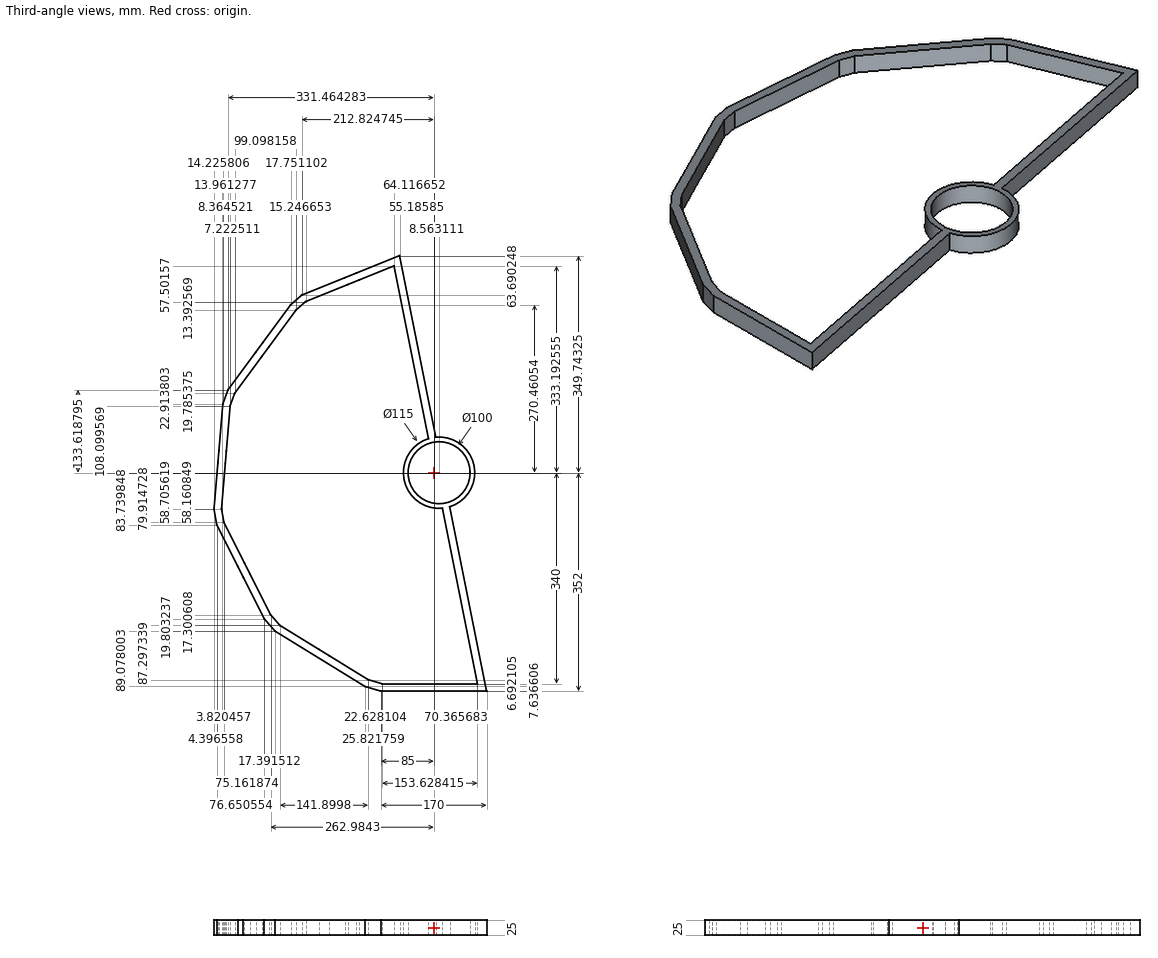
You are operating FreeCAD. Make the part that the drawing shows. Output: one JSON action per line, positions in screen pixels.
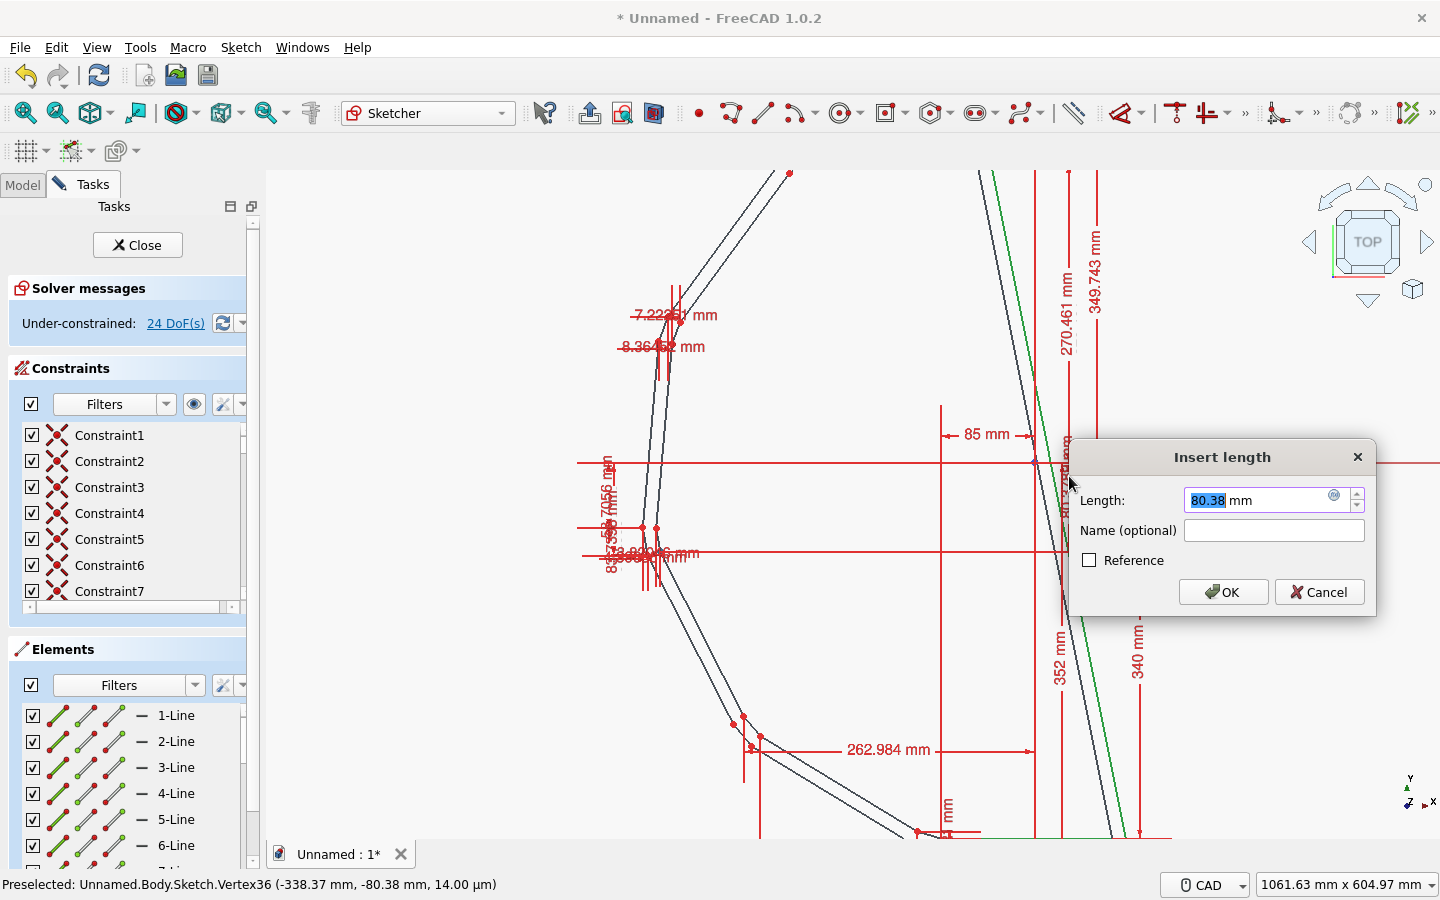
{"action": "type", "text": "79.914728"}
{"action": "key", "text": "Return"}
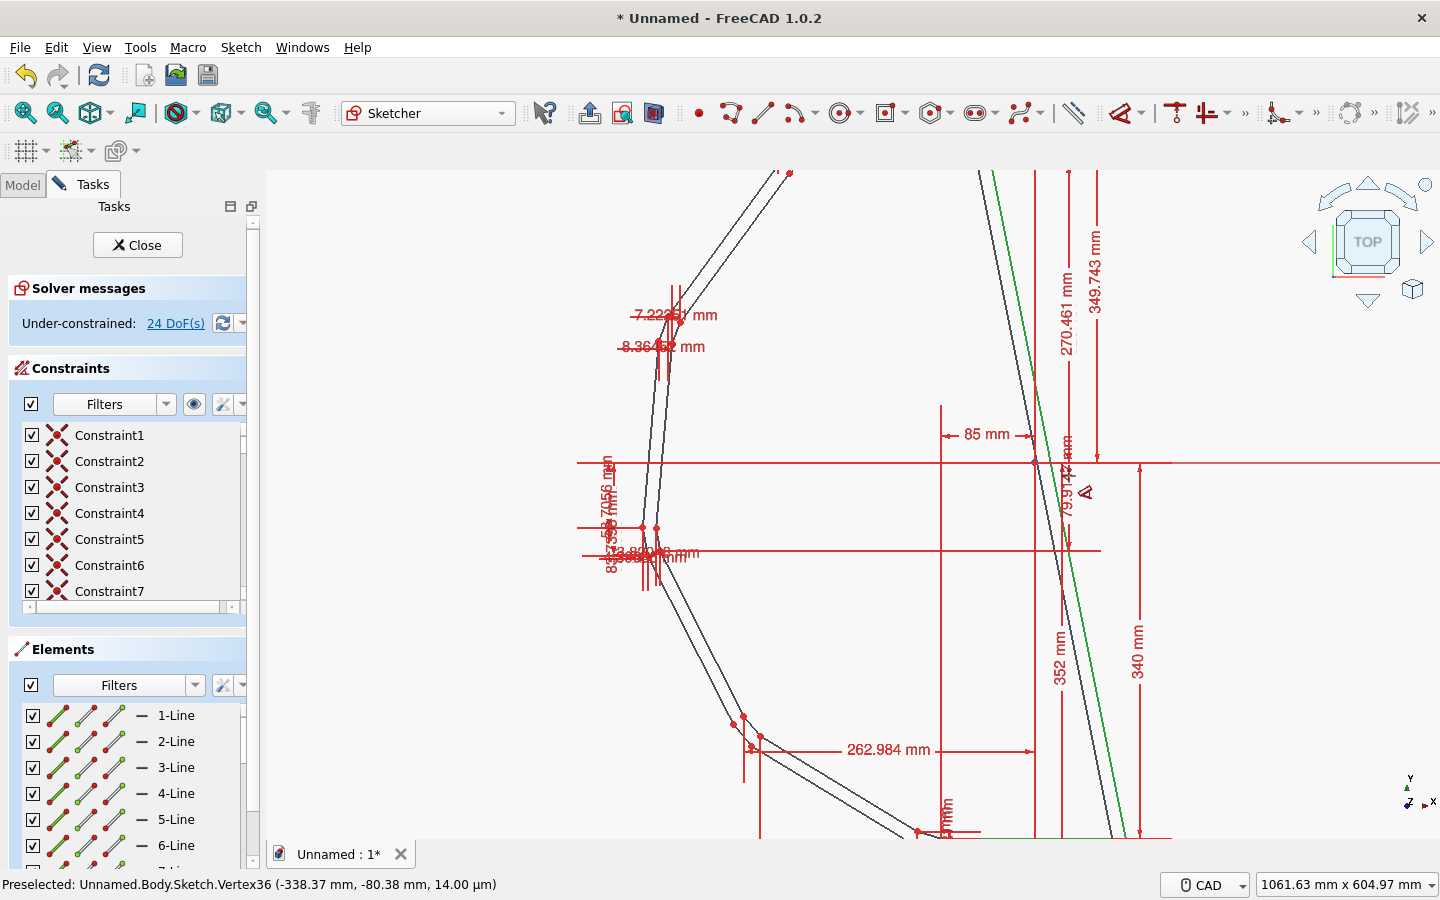
{"action": "left_click", "coordinate": [656, 528]}
{"action": "left_click", "coordinate": [1093, 511]}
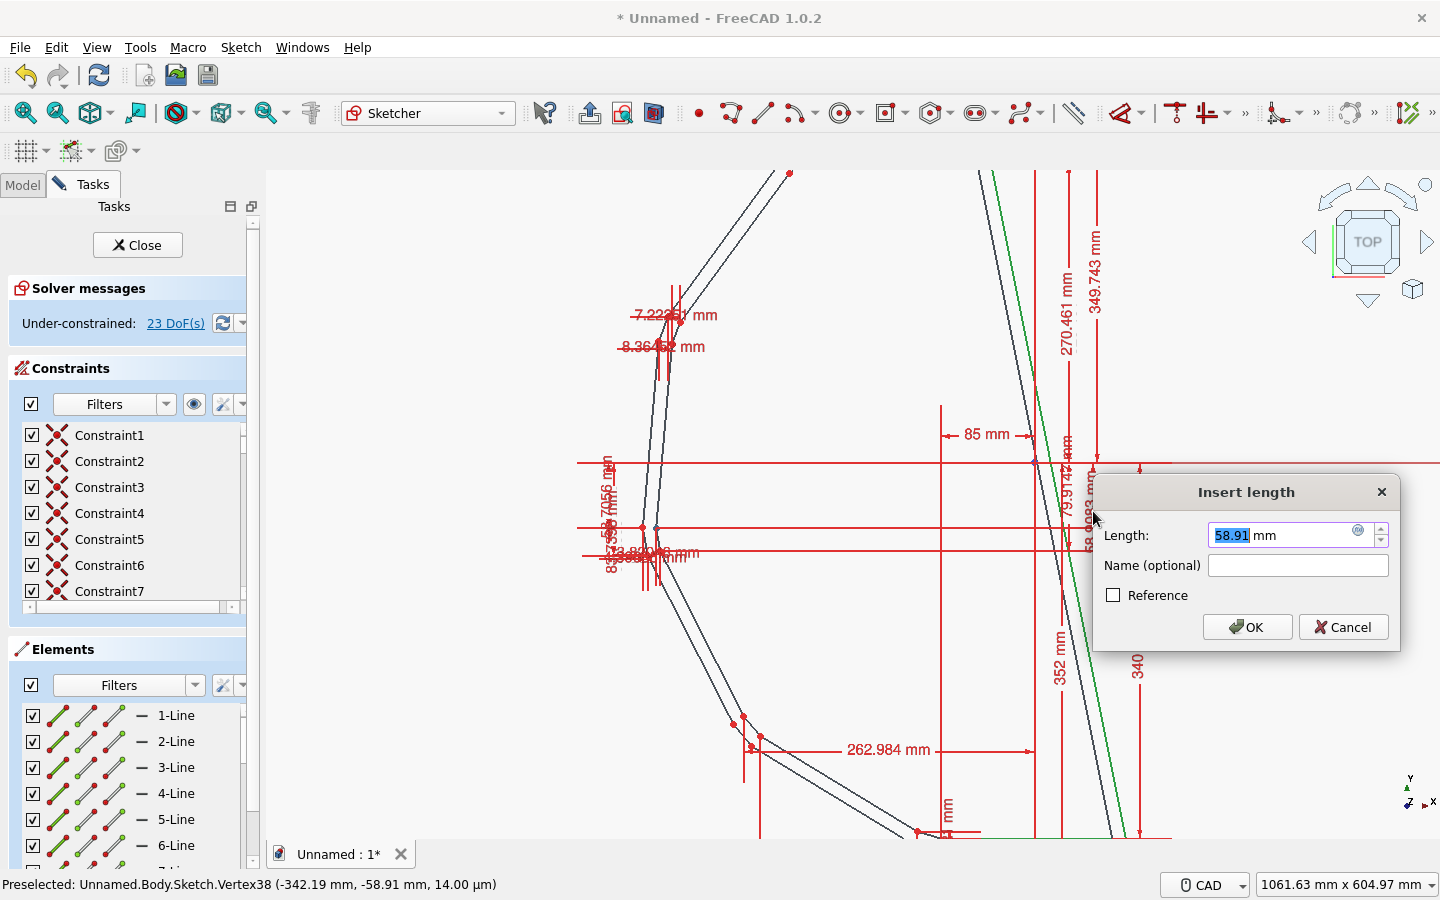
{"action": "type", "text": "58.160849"}
{"action": "key", "text": "Return"}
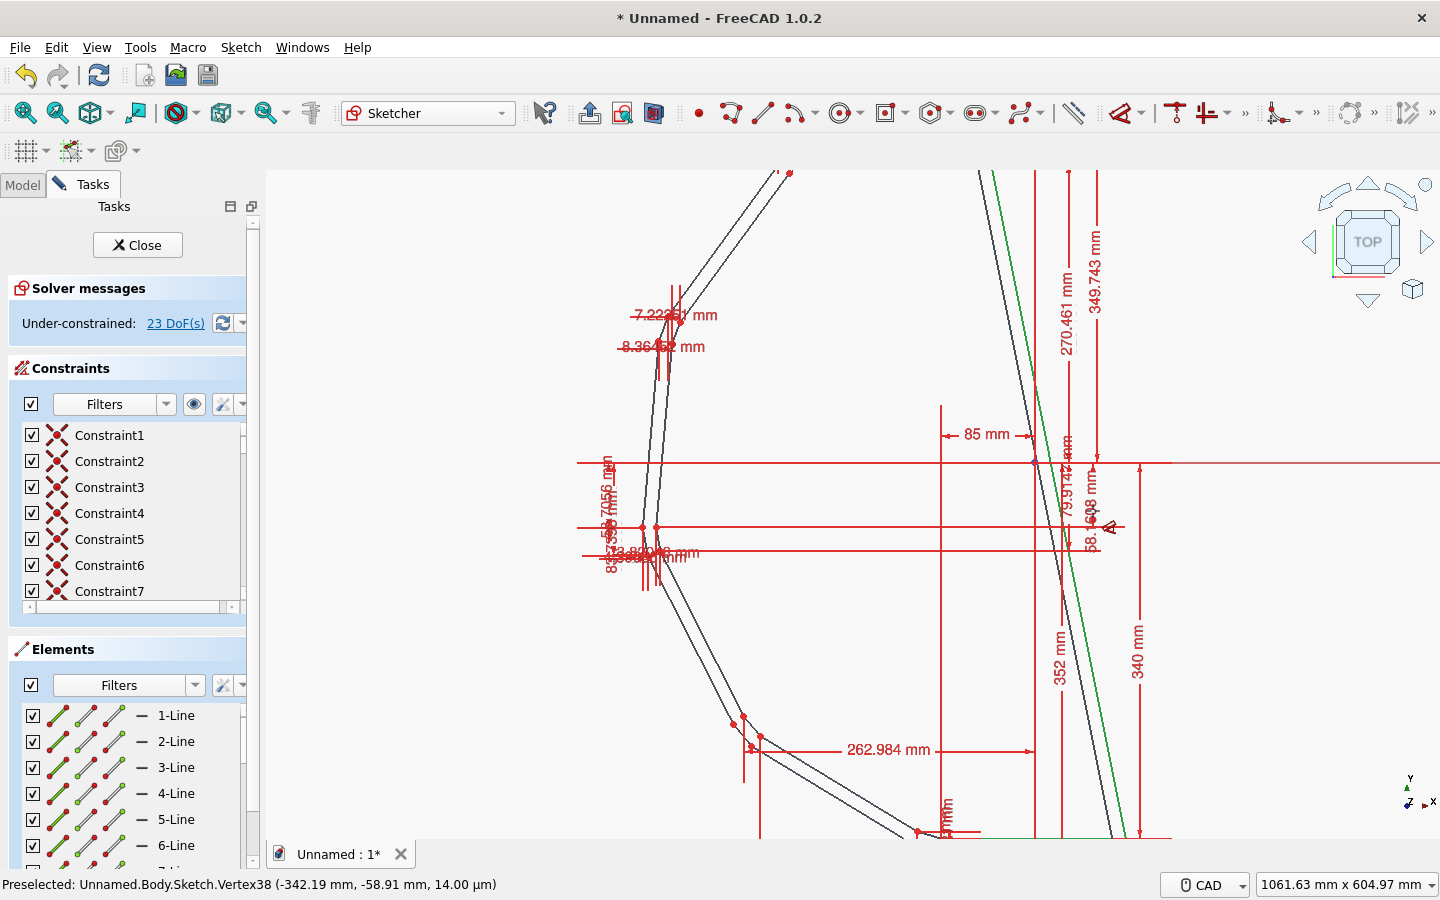
{"action": "scroll", "coordinate": [661, 553], "scroll_direction": "down", "scroll_amount": 3}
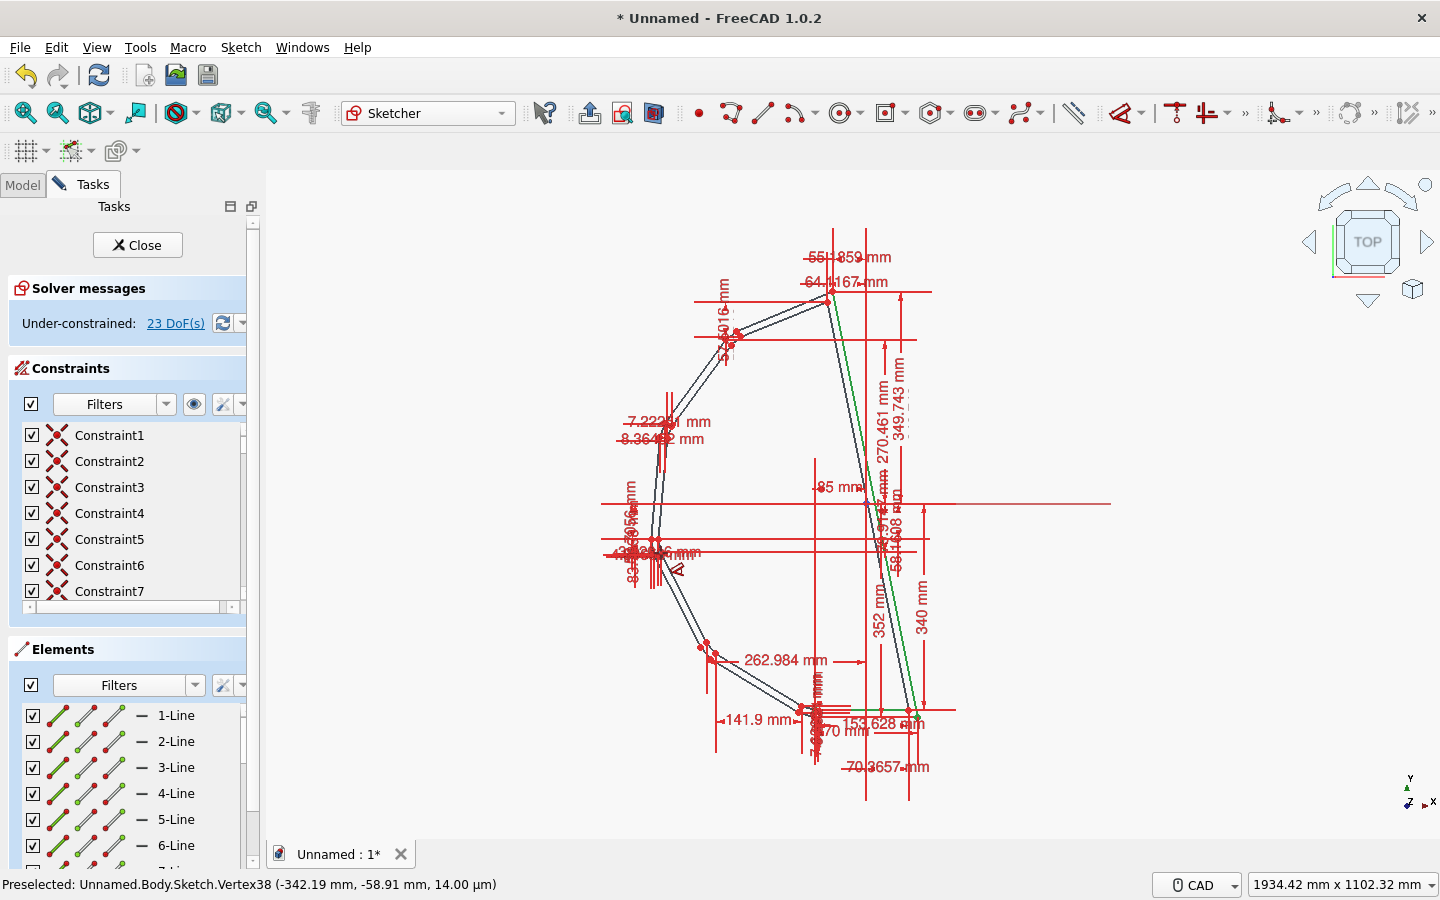
{"action": "scroll", "coordinate": [804, 304], "scroll_direction": "up", "scroll_amount": 4}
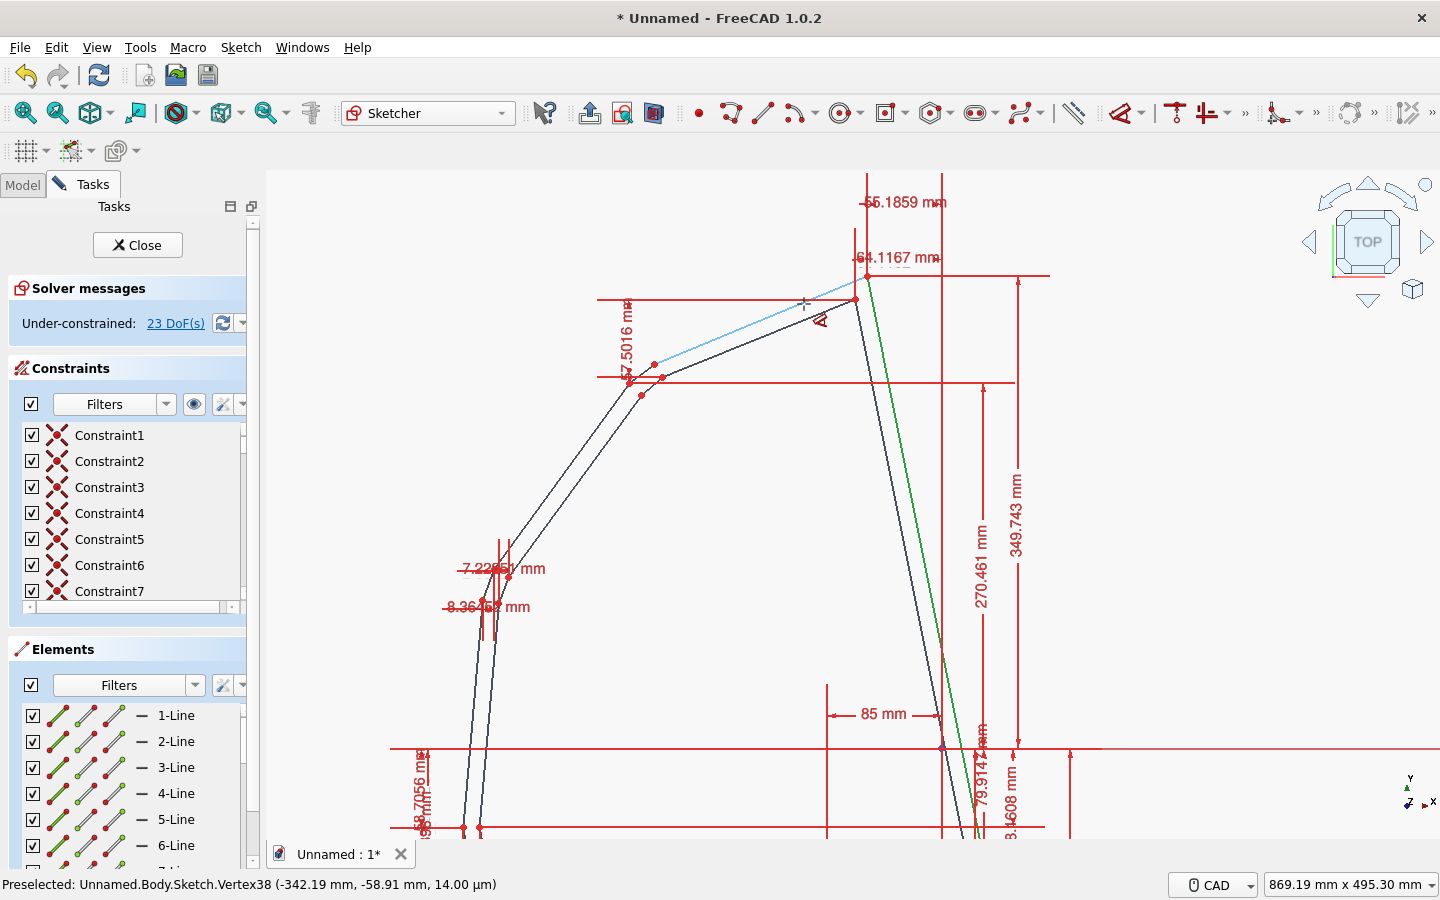
{"action": "left_click", "coordinate": [803, 303]}
{"action": "left_click", "coordinate": [901, 320]}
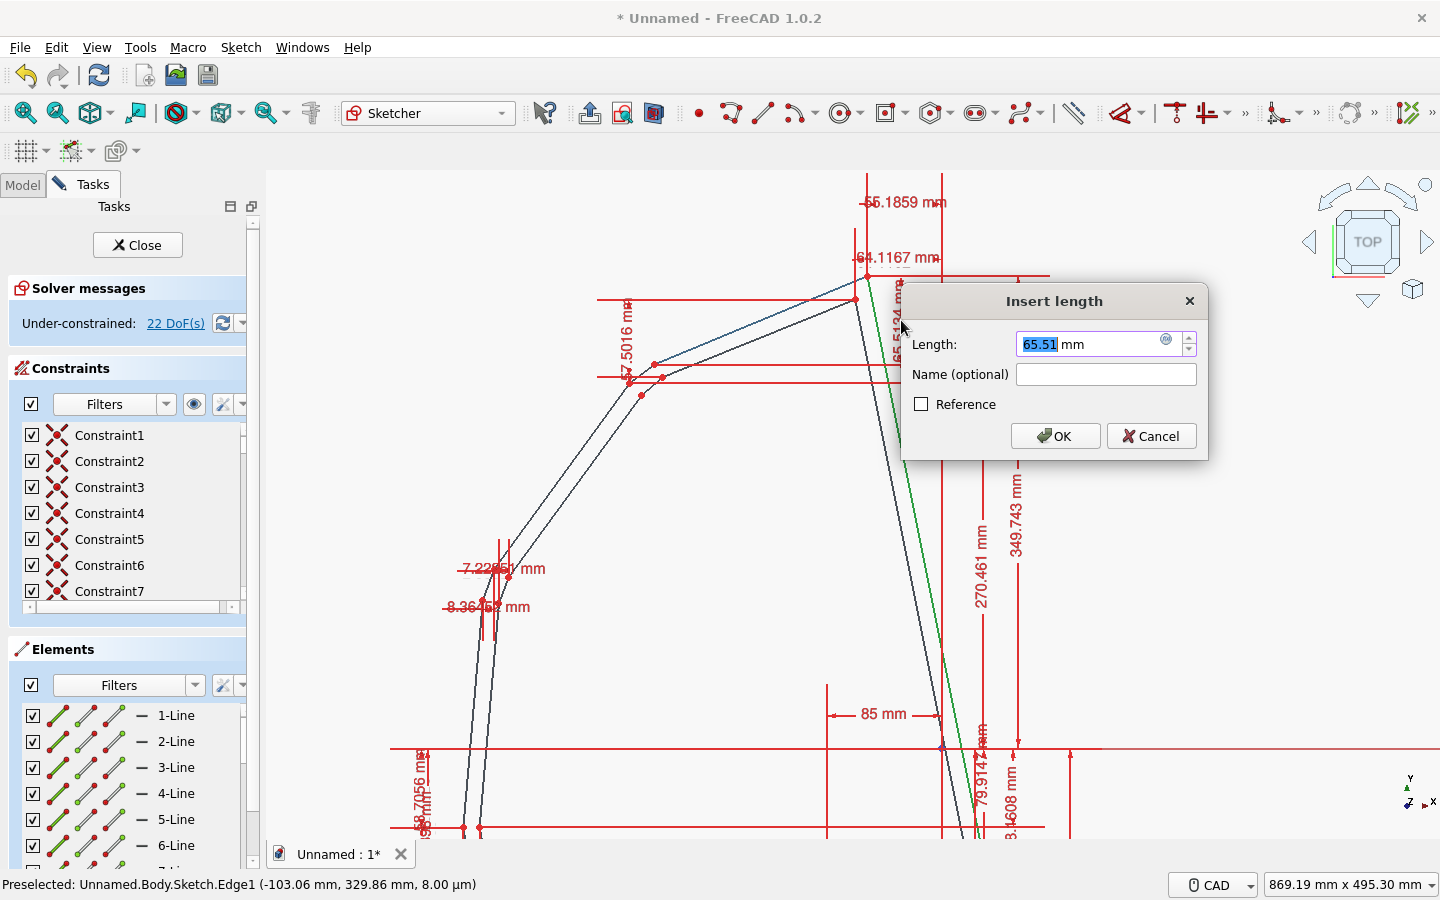
{"action": "type", "text": "63.690248"}
{"action": "key", "text": "Return"}